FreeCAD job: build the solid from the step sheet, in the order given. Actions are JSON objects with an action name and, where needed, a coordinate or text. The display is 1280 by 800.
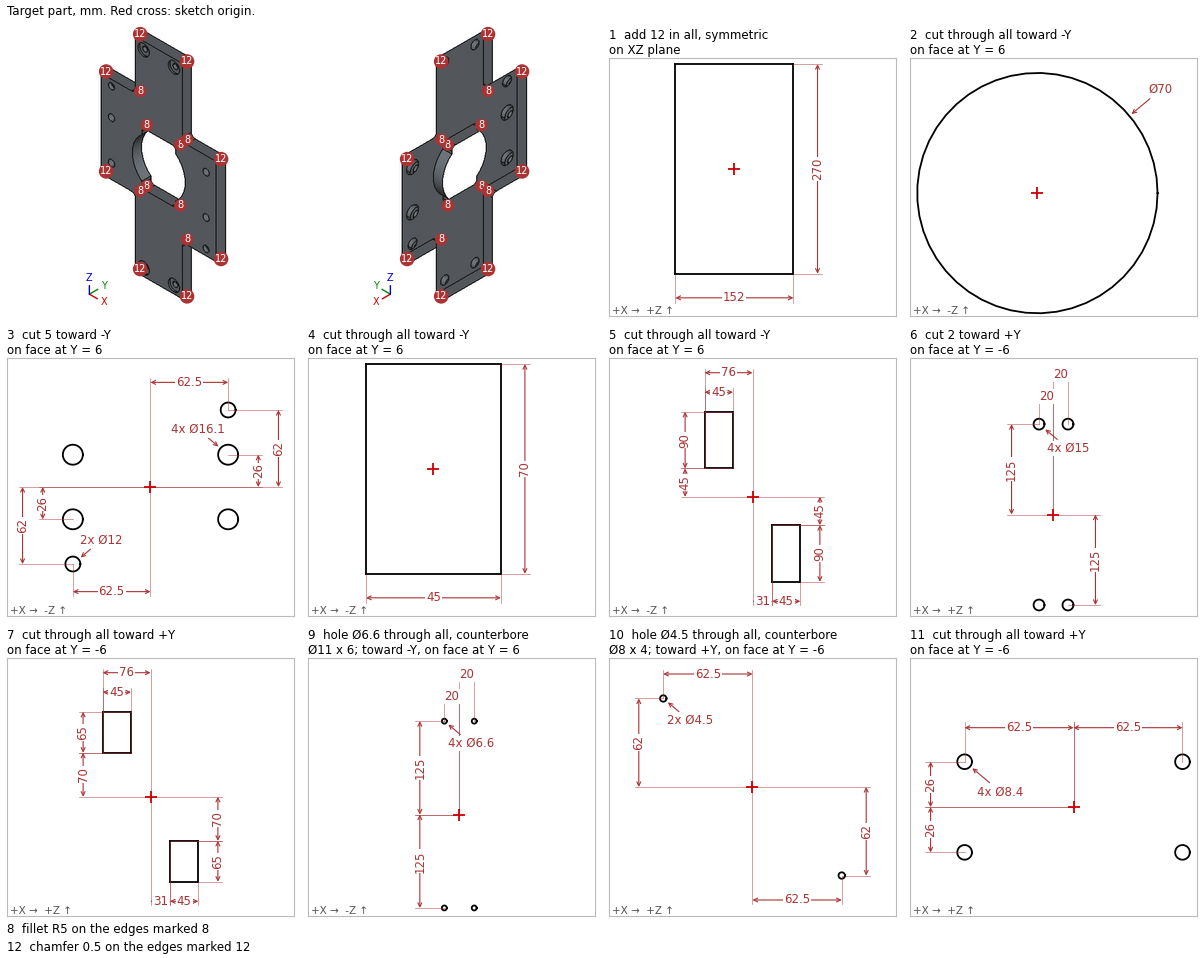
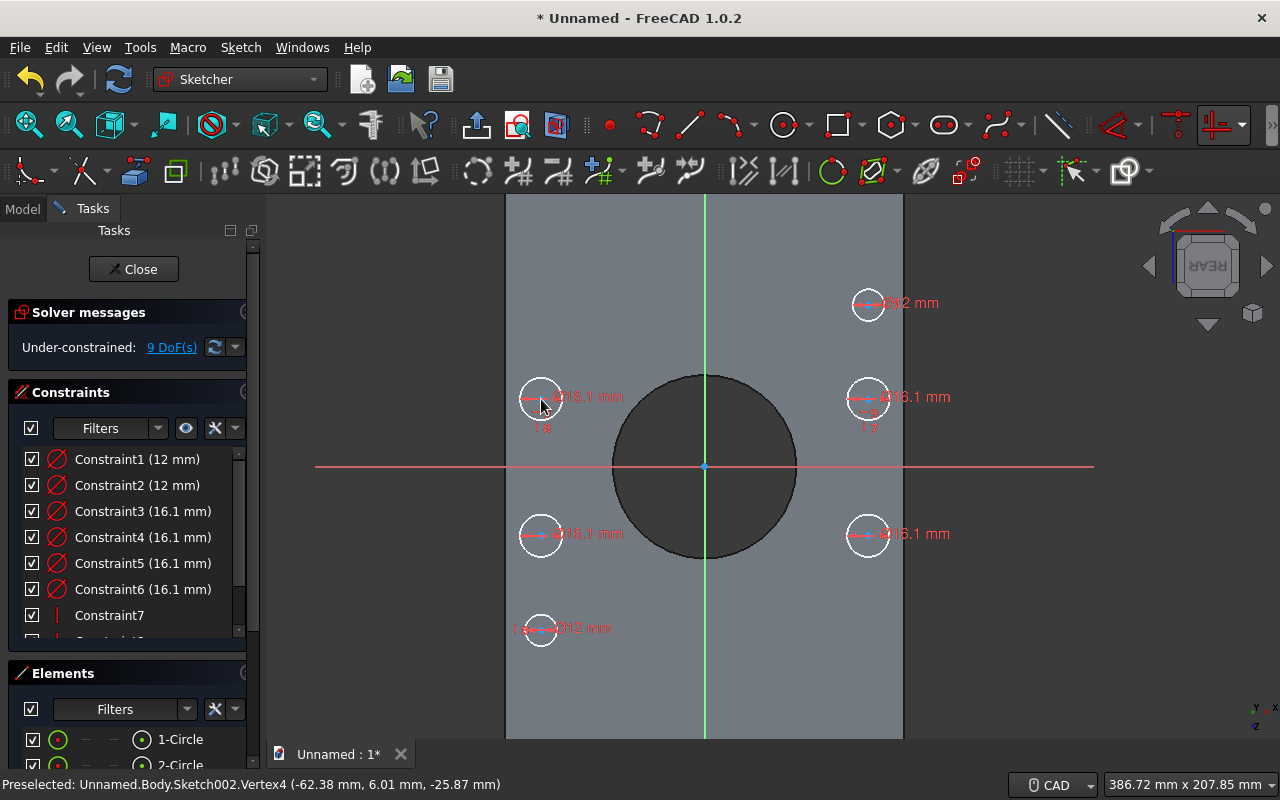
{"action": "left_click", "coordinate": [541, 630]}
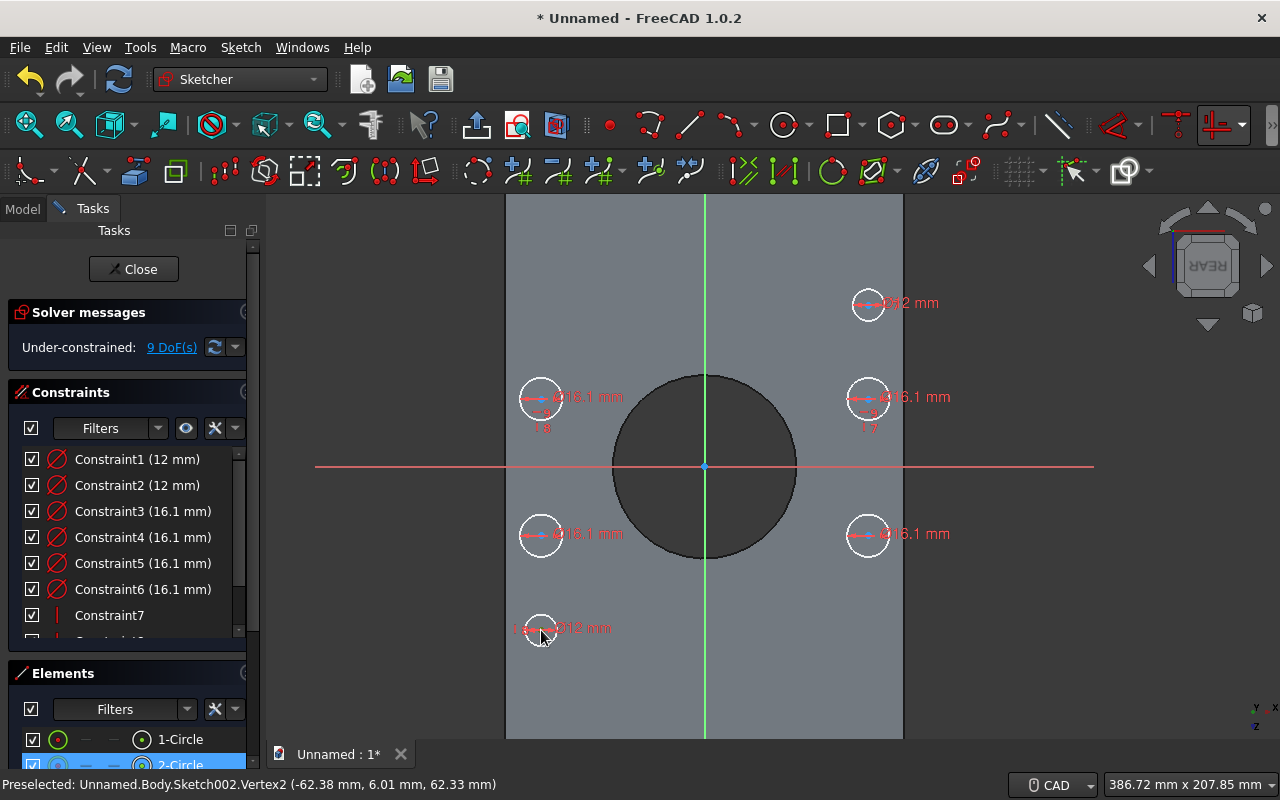
{"action": "left_click", "coordinate": [541, 536]}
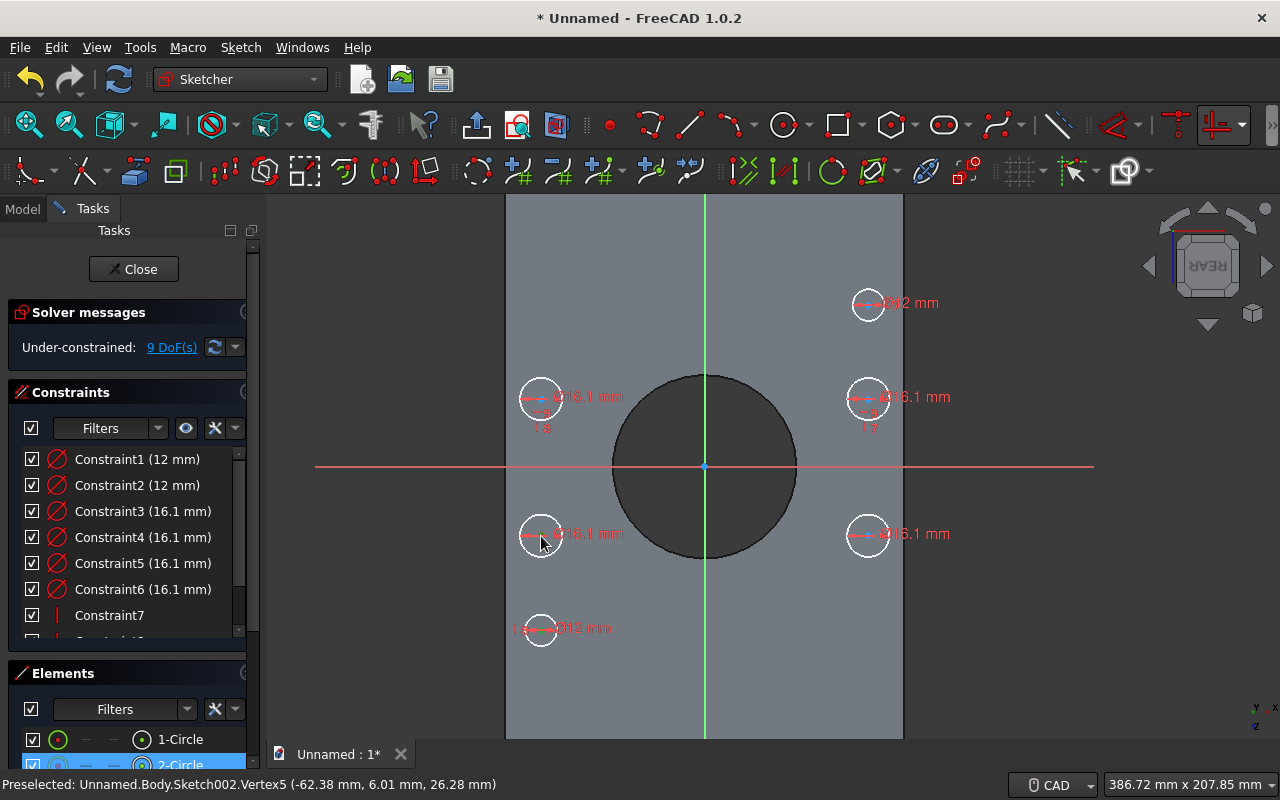
{"action": "key", "text": "v"}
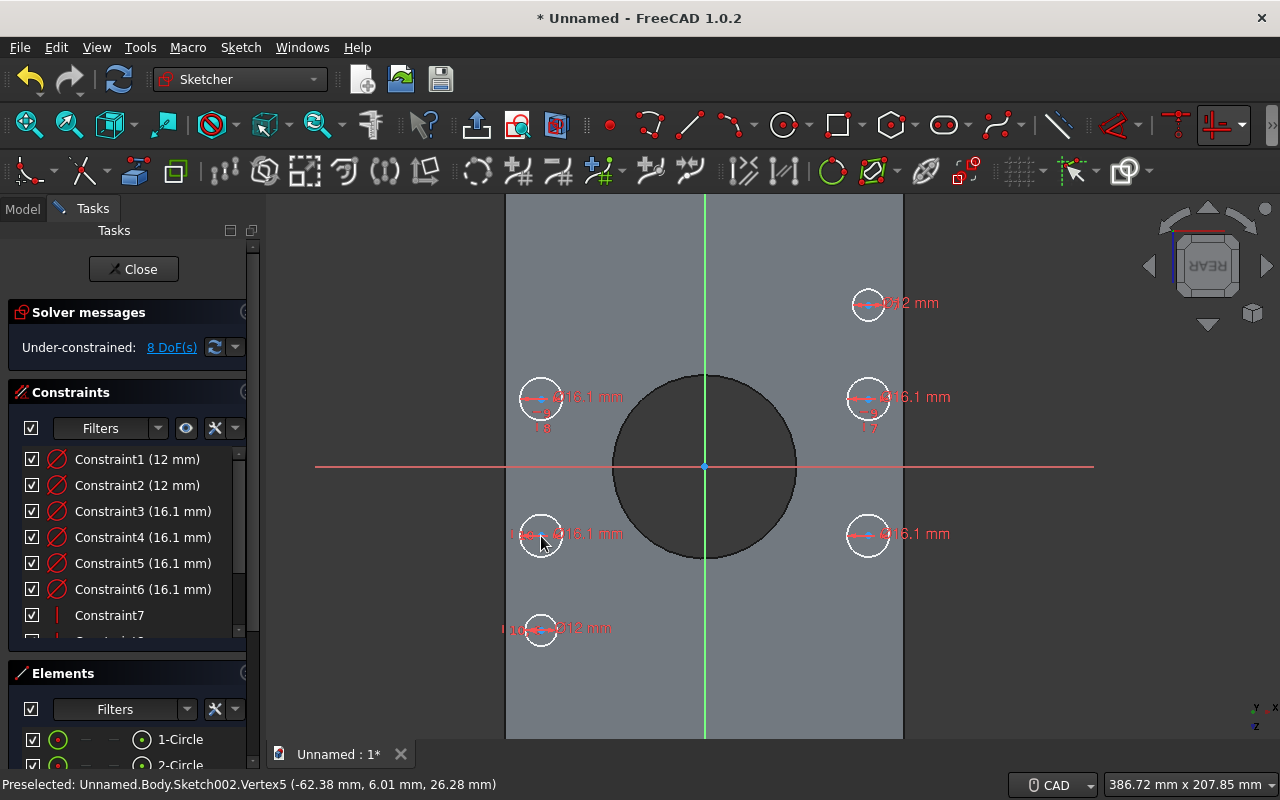
{"action": "left_click", "coordinate": [869, 399]}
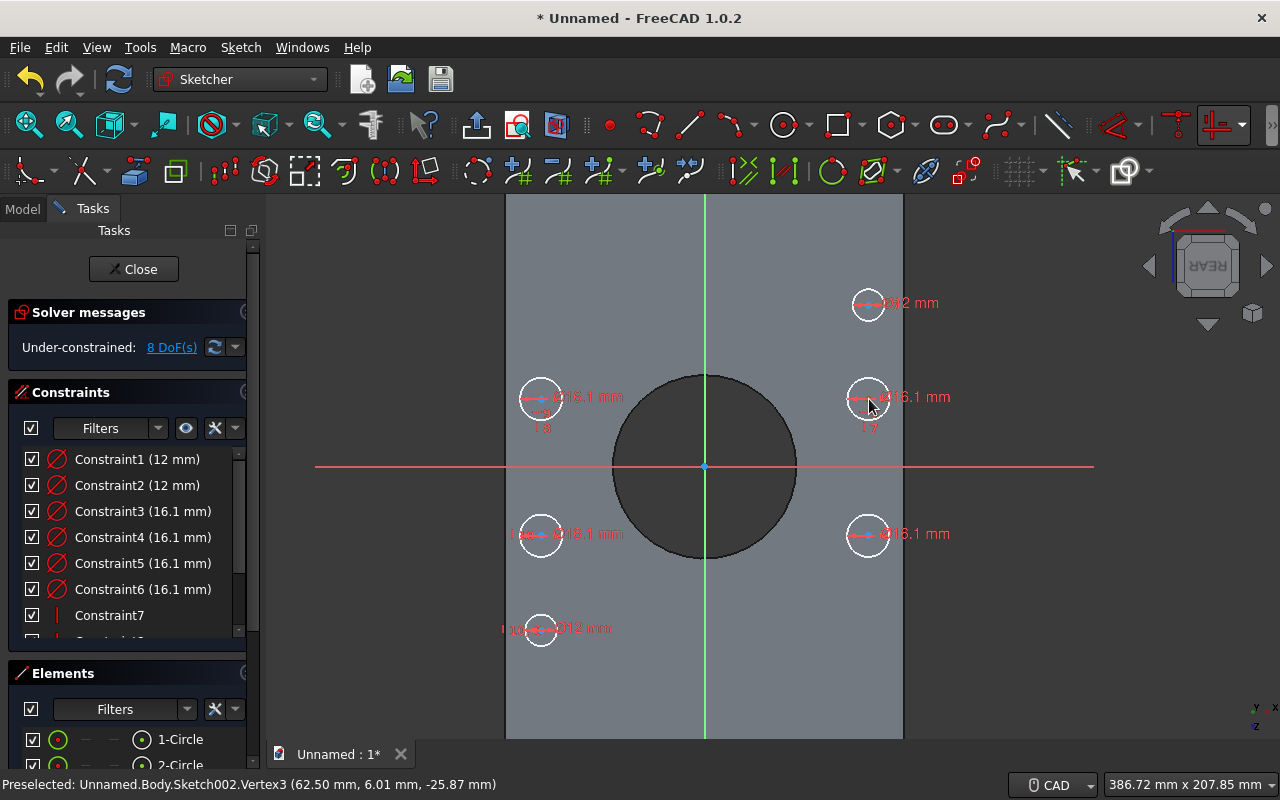
{"action": "left_click", "coordinate": [868, 536]}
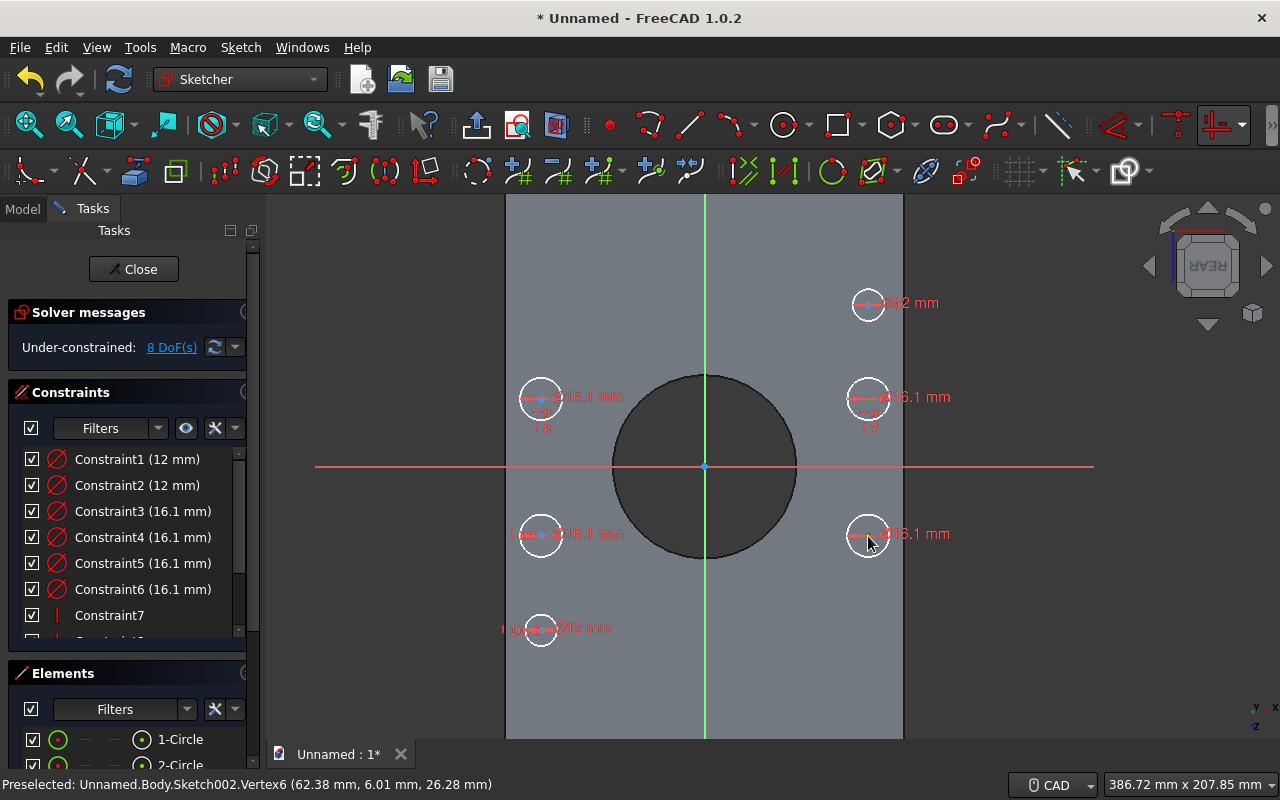
{"action": "key", "text": "v"}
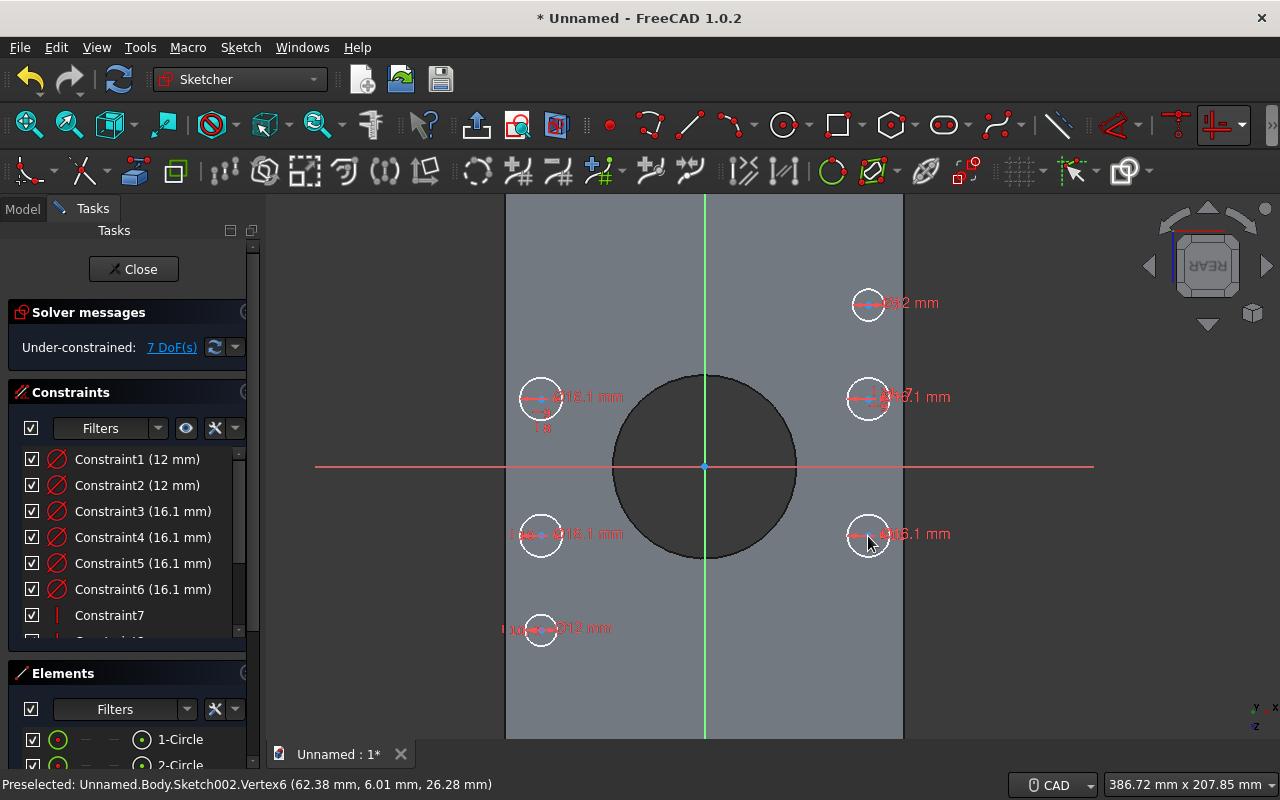
{"action": "left_click", "coordinate": [541, 536]}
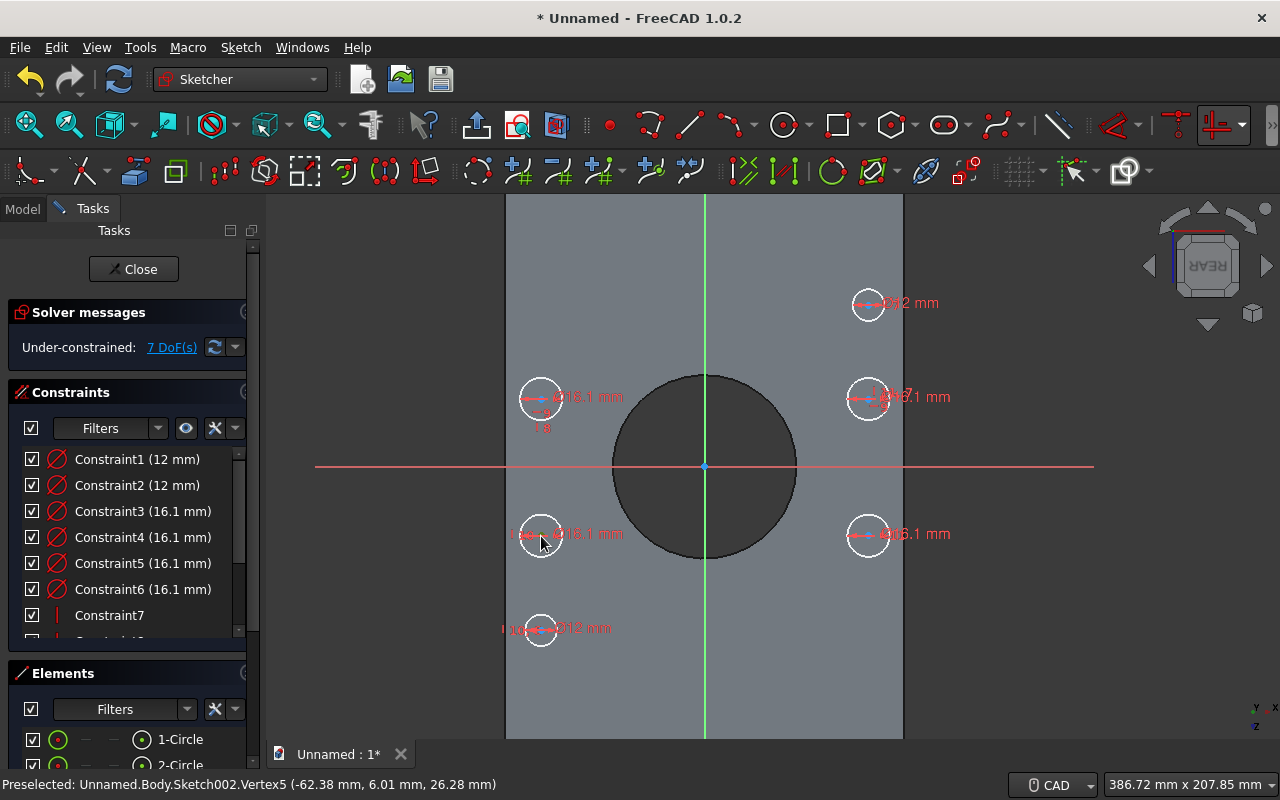
{"action": "left_click", "coordinate": [869, 536]}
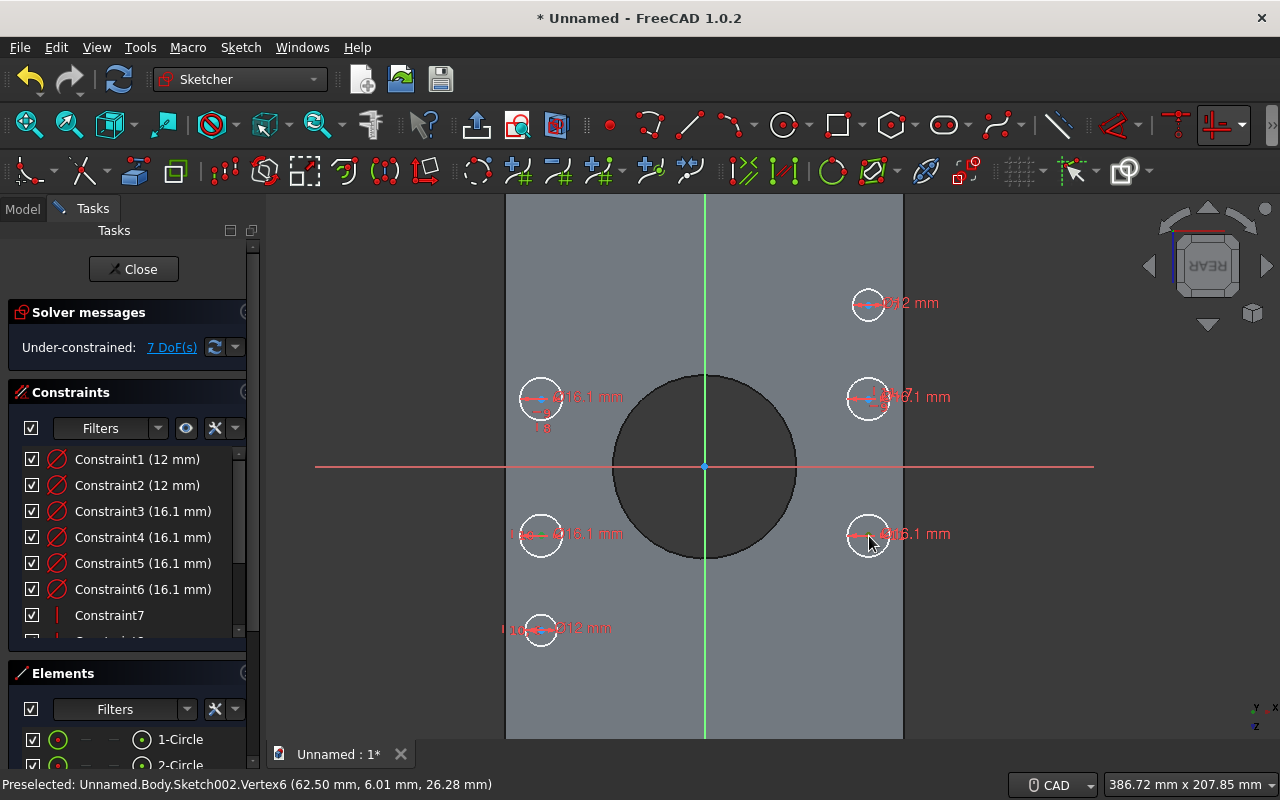
{"action": "left_click", "coordinate": [1244, 126]}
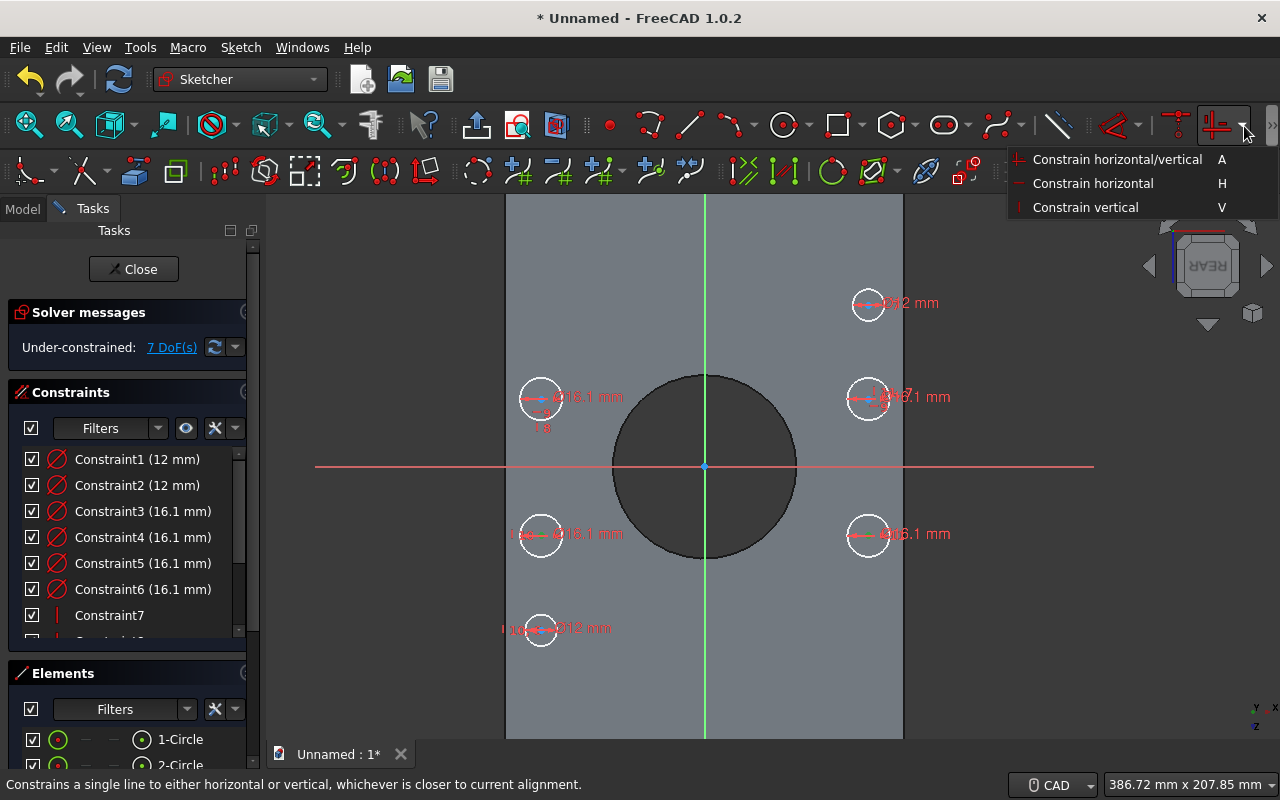
{"action": "left_click", "coordinate": [1143, 183]}